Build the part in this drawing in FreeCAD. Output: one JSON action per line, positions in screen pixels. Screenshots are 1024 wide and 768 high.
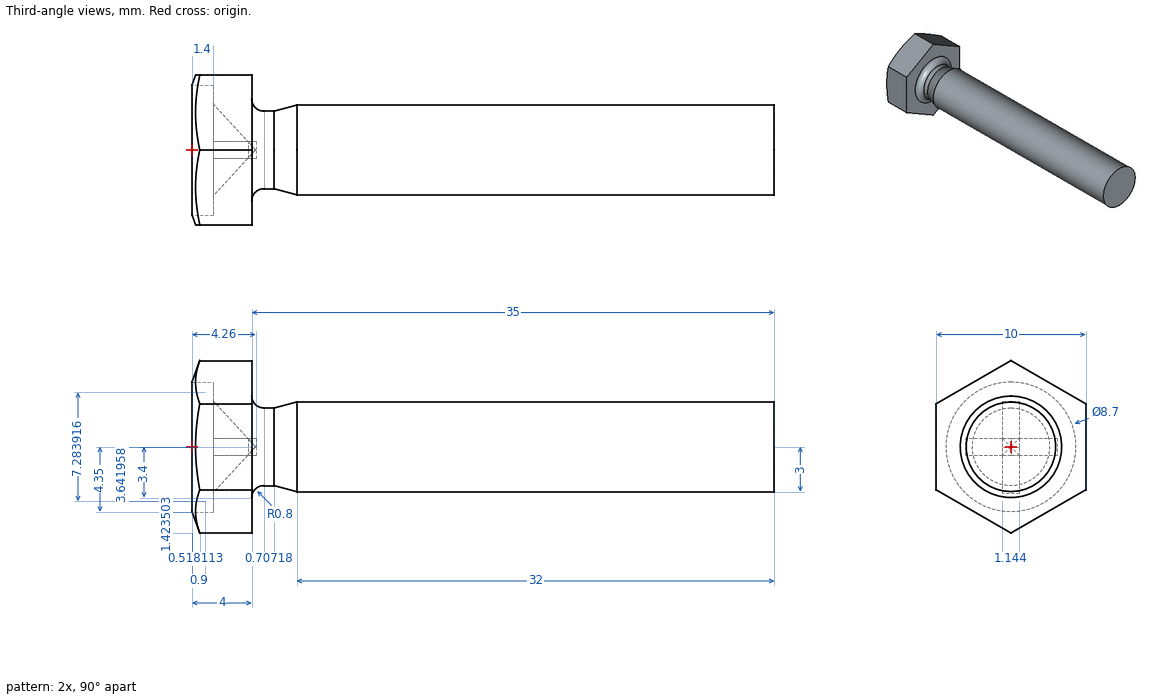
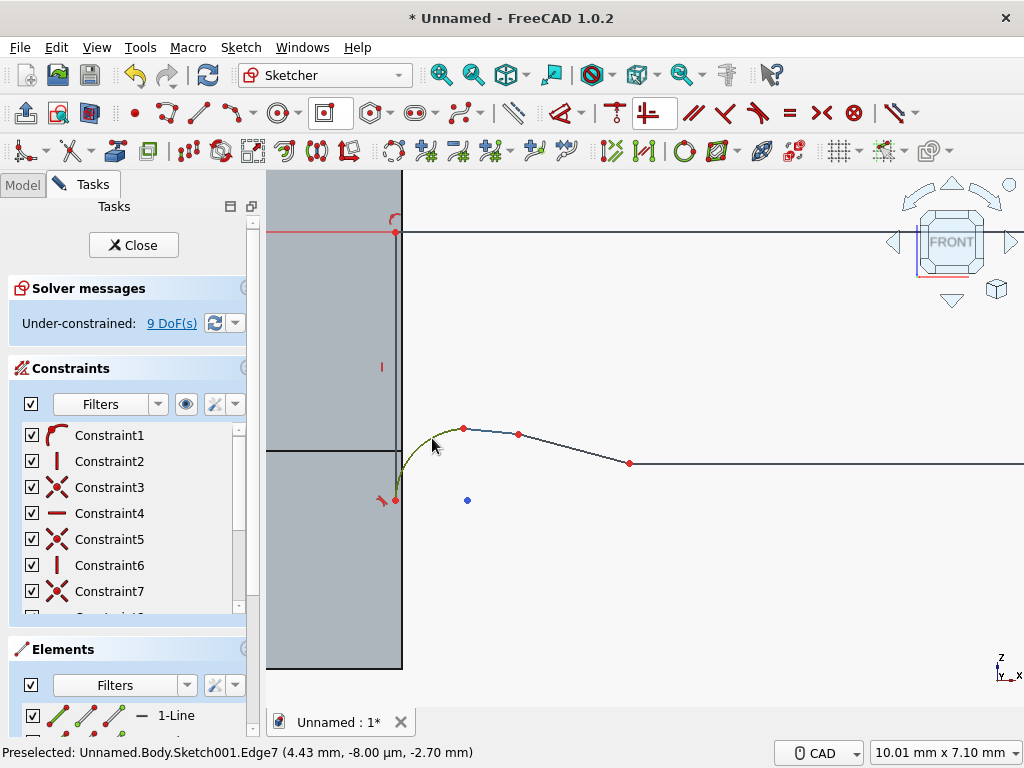
{"action": "left_click", "coordinate": [758, 114]}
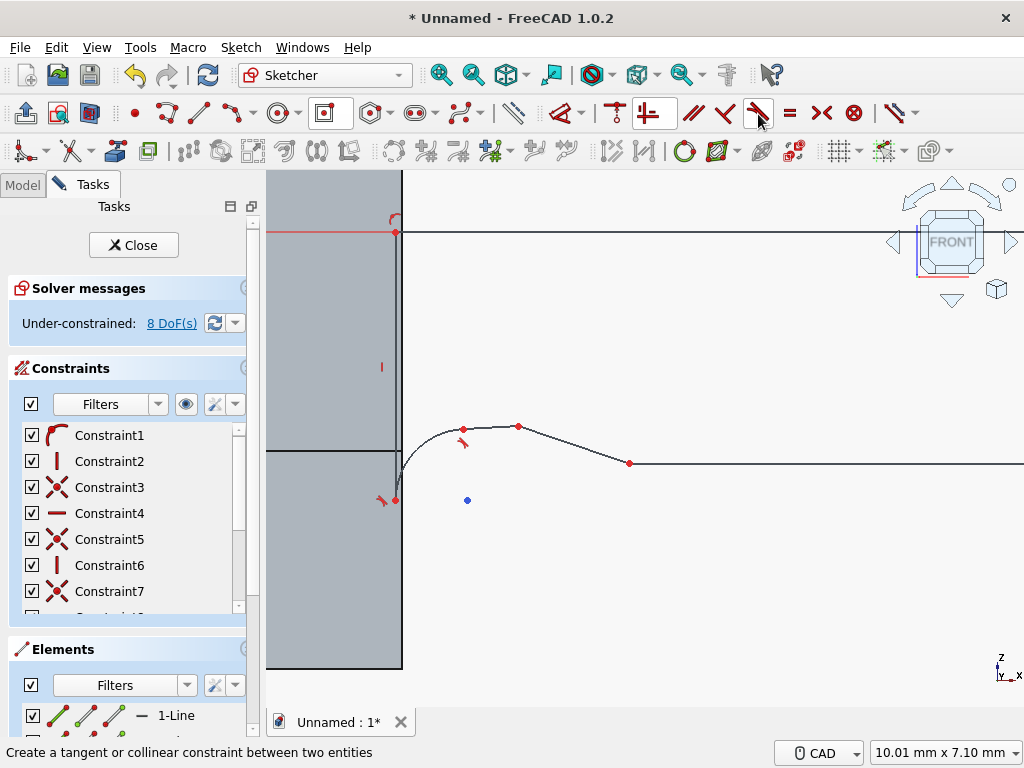
{"action": "left_click", "coordinate": [502, 427]}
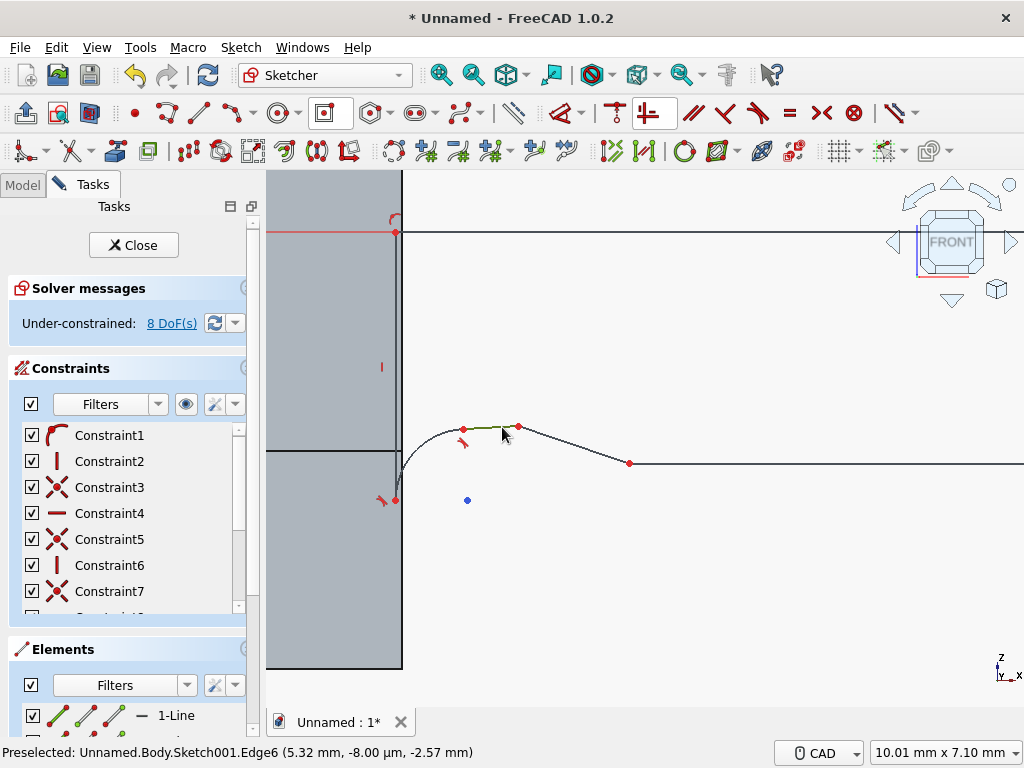
{"action": "left_click", "coordinate": [672, 114]}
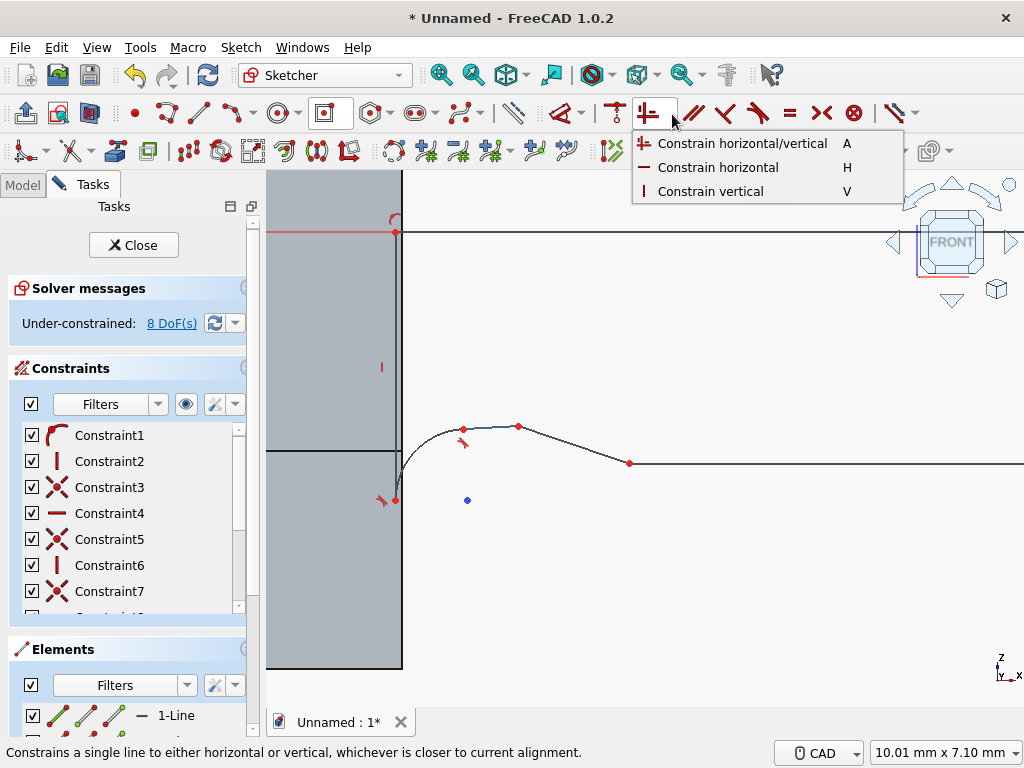
{"action": "left_click", "coordinate": [768, 167]}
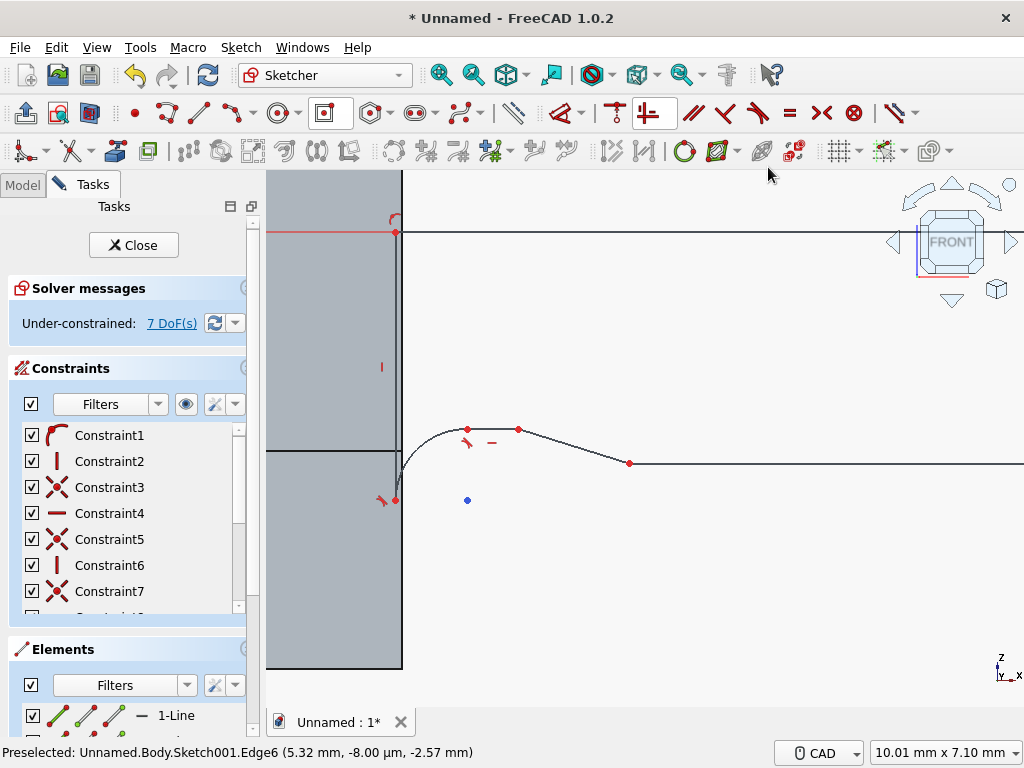
{"action": "left_click", "coordinate": [435, 437]}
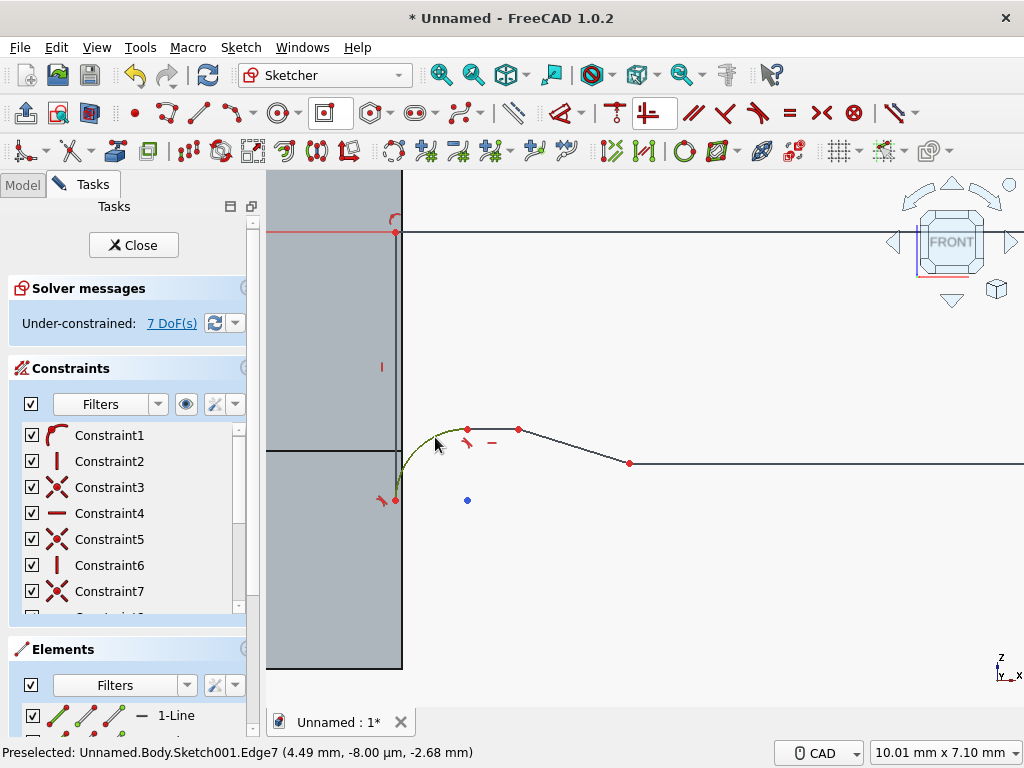
{"action": "key", "text": "k r"}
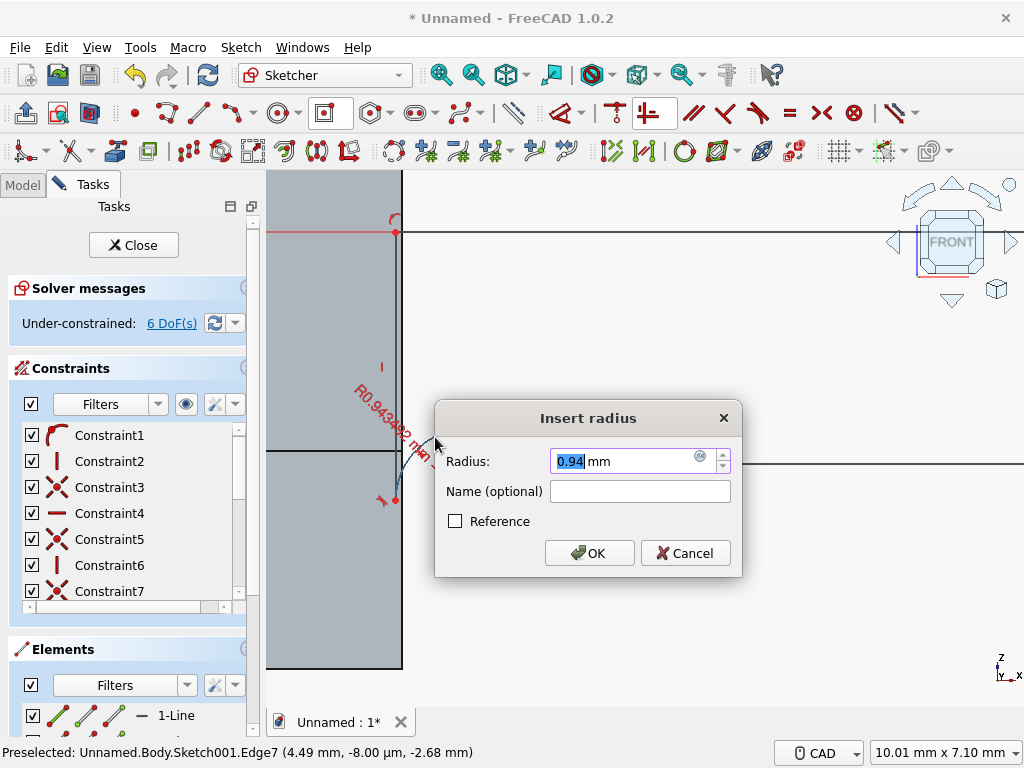
{"action": "type", "text": "0.8"}
{"action": "key", "text": "Return"}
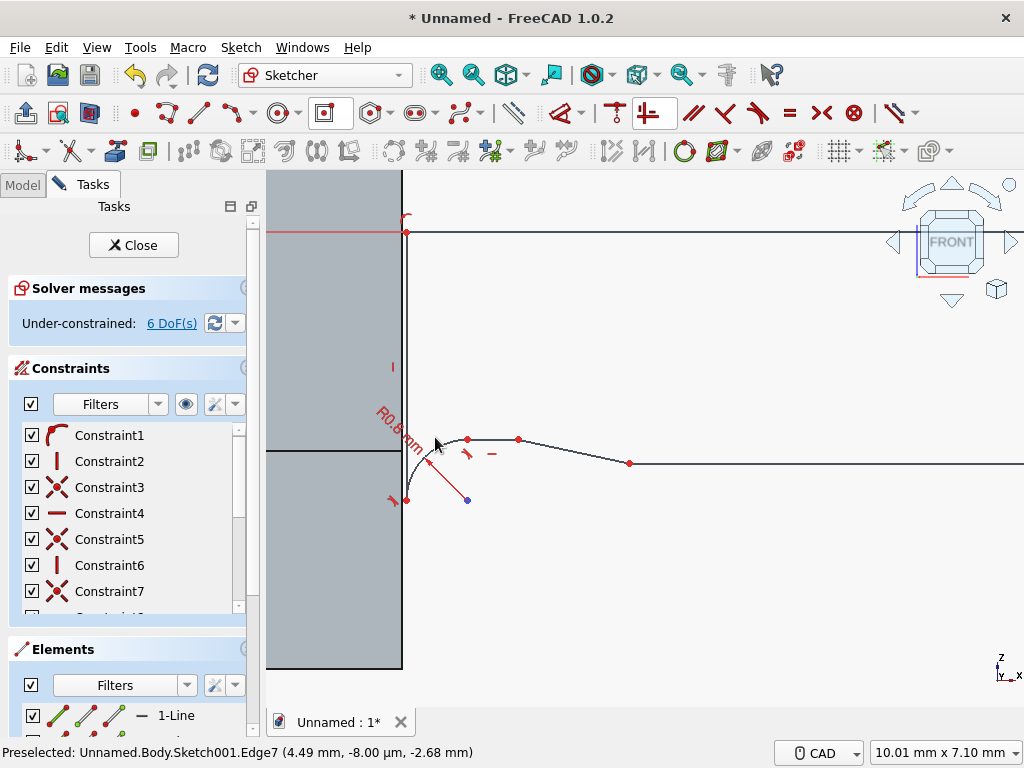
{"action": "scroll", "coordinate": [420, 451], "scroll_direction": "down", "scroll_amount": 10}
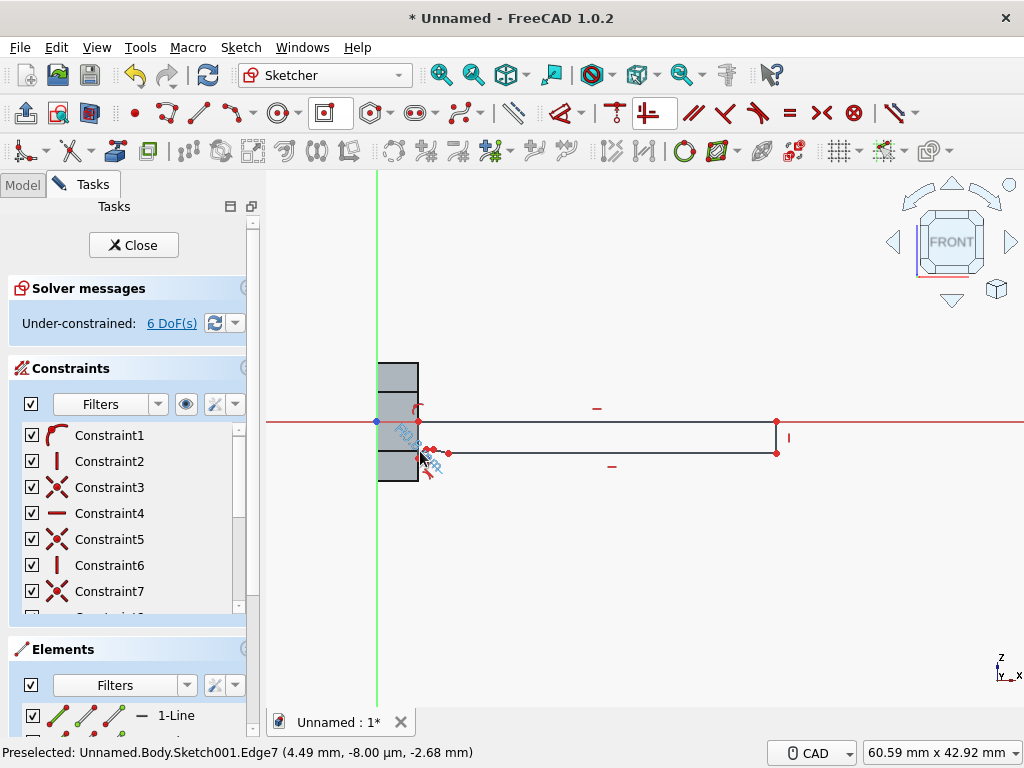
{"action": "scroll", "coordinate": [776, 431], "scroll_direction": "up", "scroll_amount": 2}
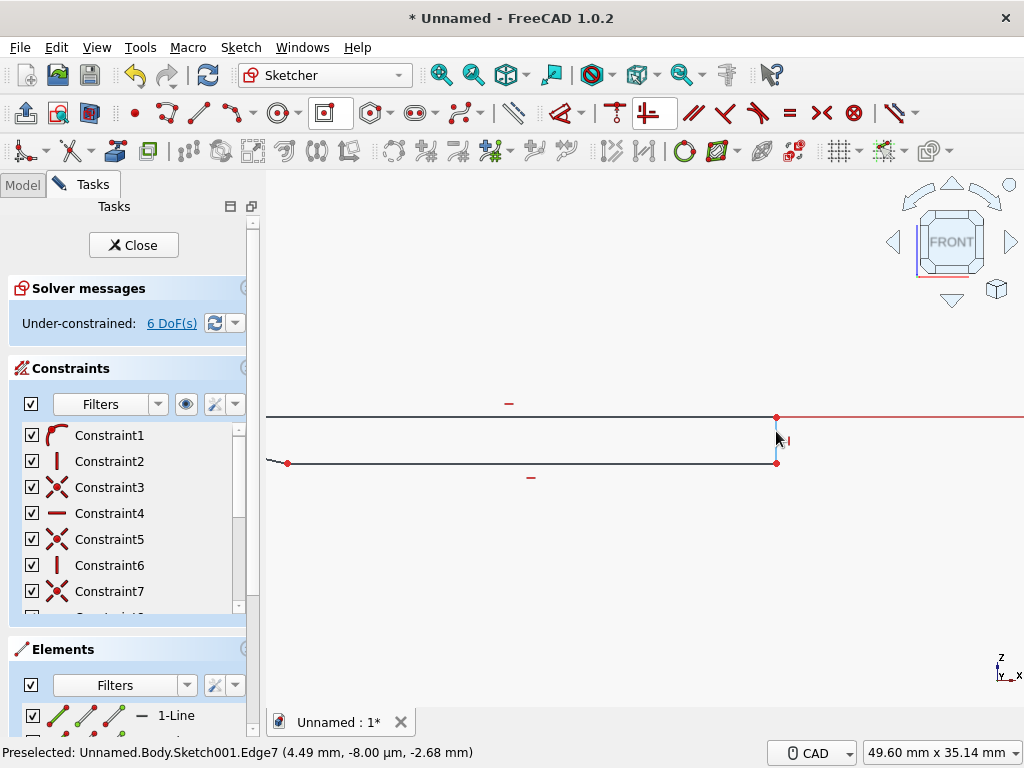
{"action": "left_click", "coordinate": [776, 431]}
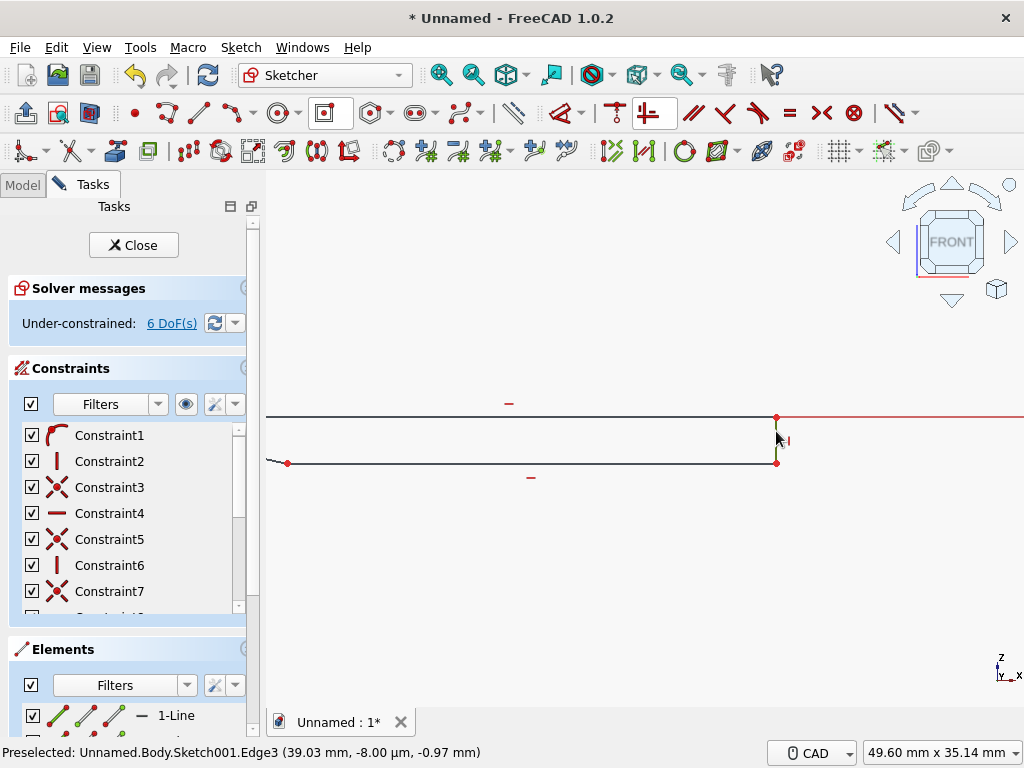
{"action": "left_click", "coordinate": [584, 114]}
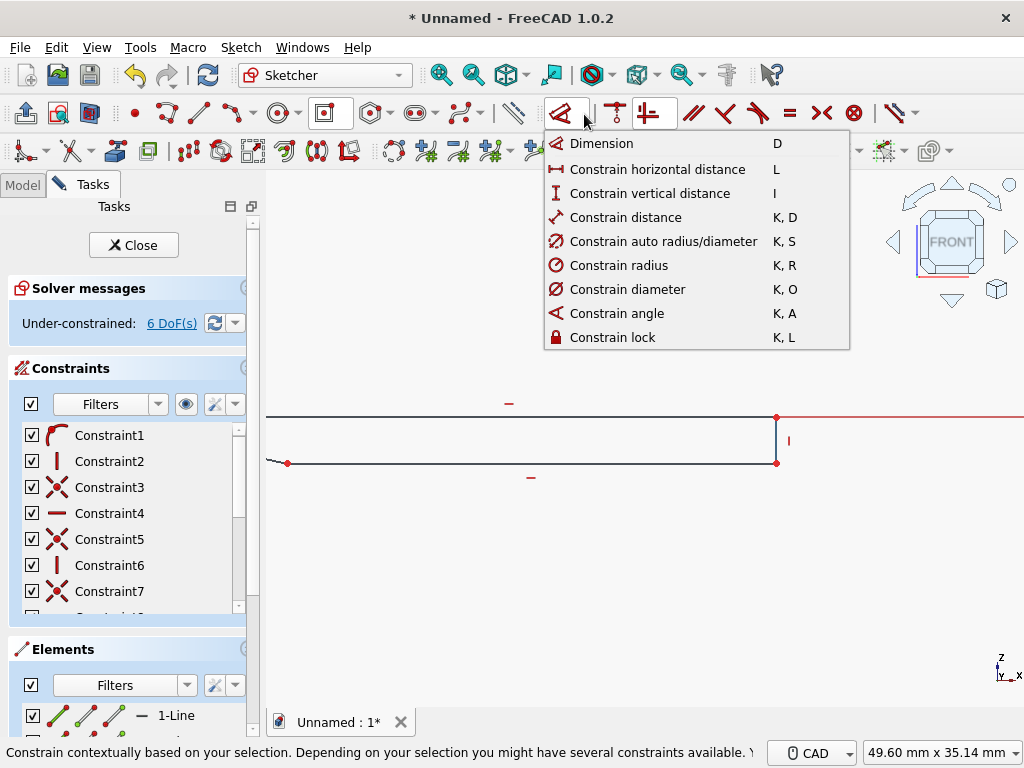
{"action": "left_click", "coordinate": [697, 193]}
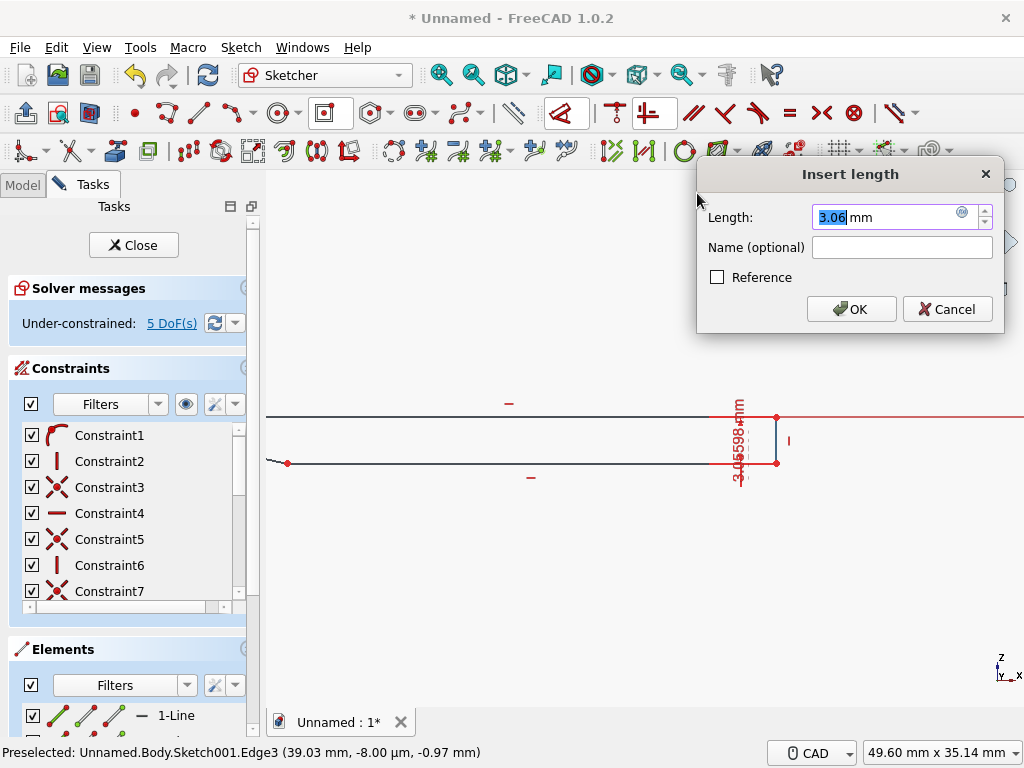
{"action": "type", "text": "3"}
{"action": "key", "text": "Return"}